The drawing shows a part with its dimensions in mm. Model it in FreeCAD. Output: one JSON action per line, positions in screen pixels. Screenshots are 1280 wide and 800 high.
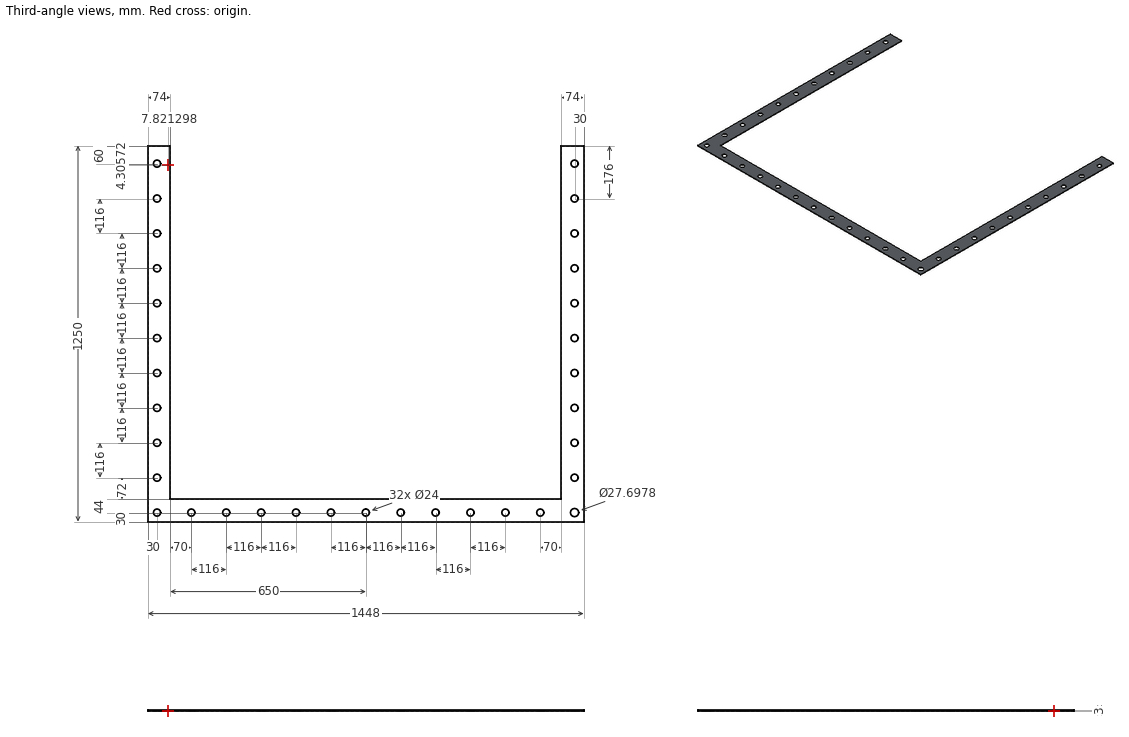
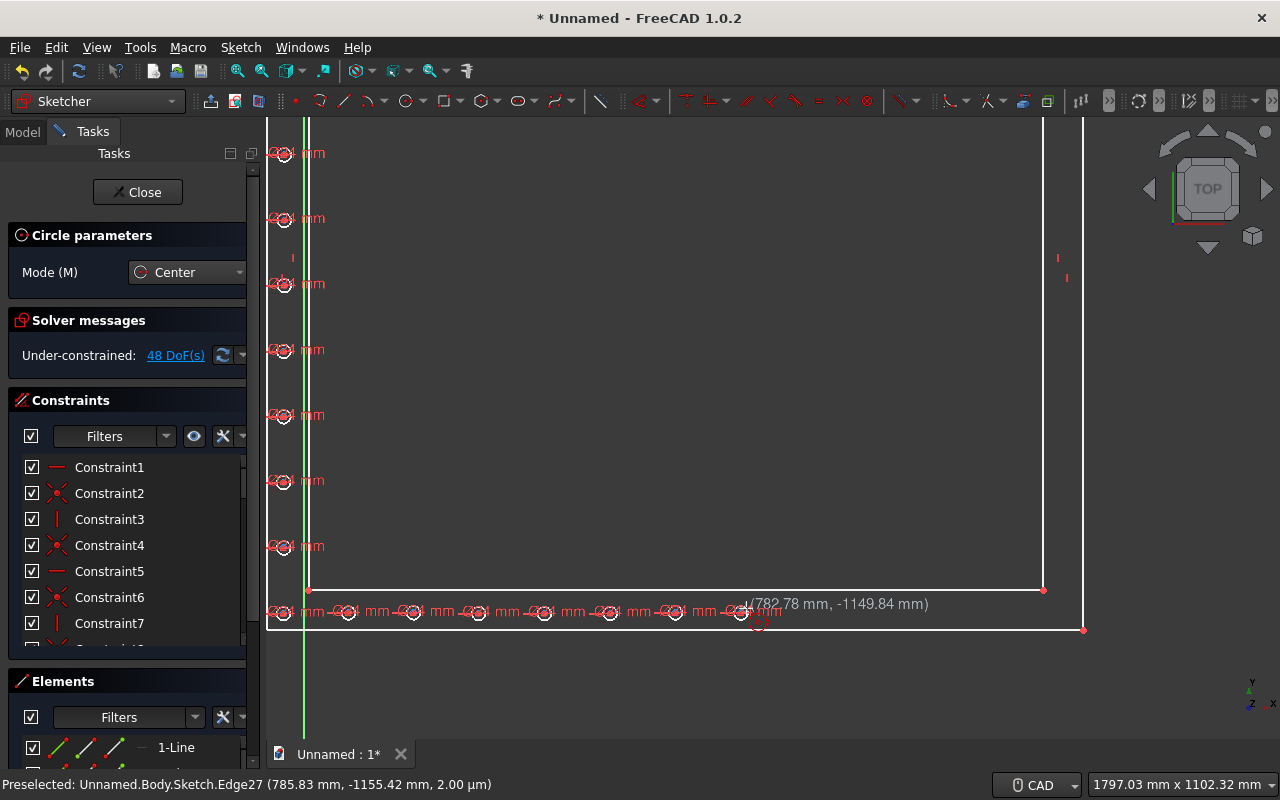
{"action": "scroll", "coordinate": [806, 612], "scroll_direction": "up", "scroll_amount": 7}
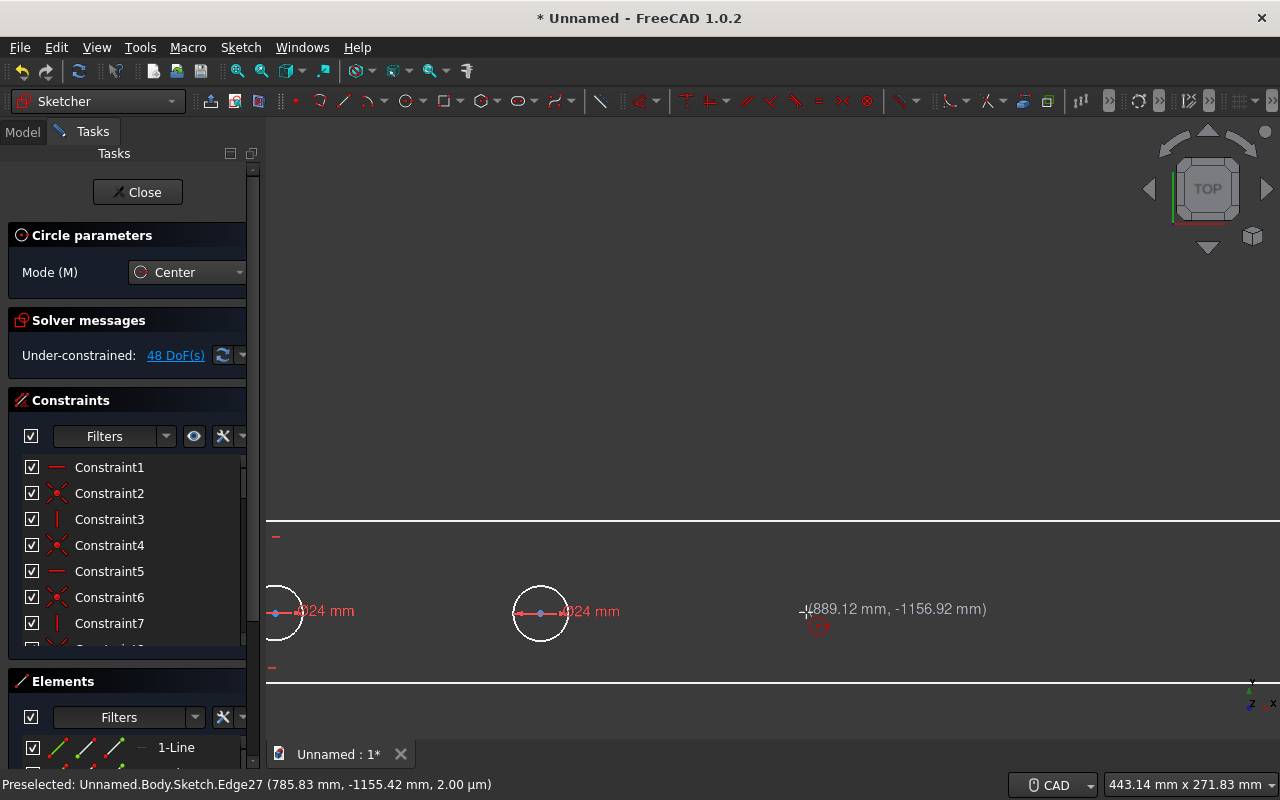
{"action": "scroll", "coordinate": [772, 612], "scroll_direction": "down", "scroll_amount": 10}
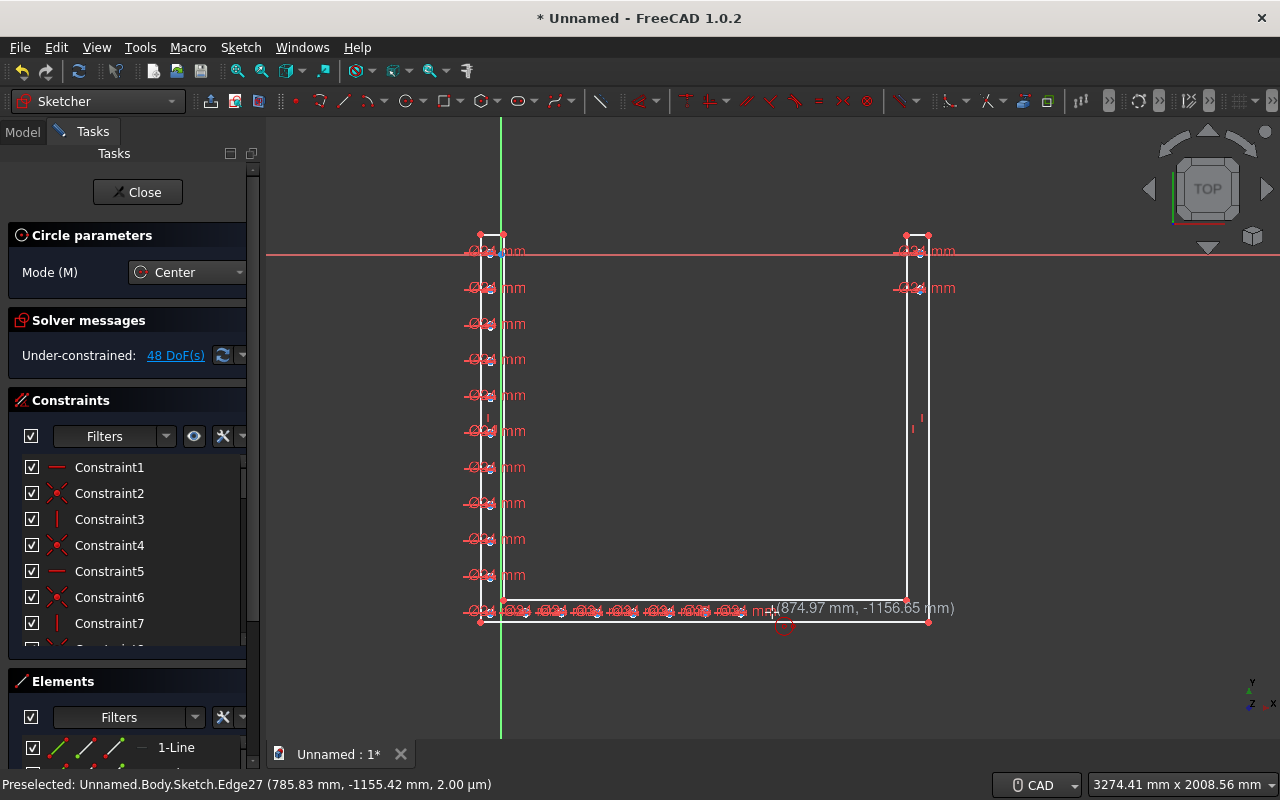
{"action": "scroll", "coordinate": [777, 613], "scroll_direction": "up", "scroll_amount": 3}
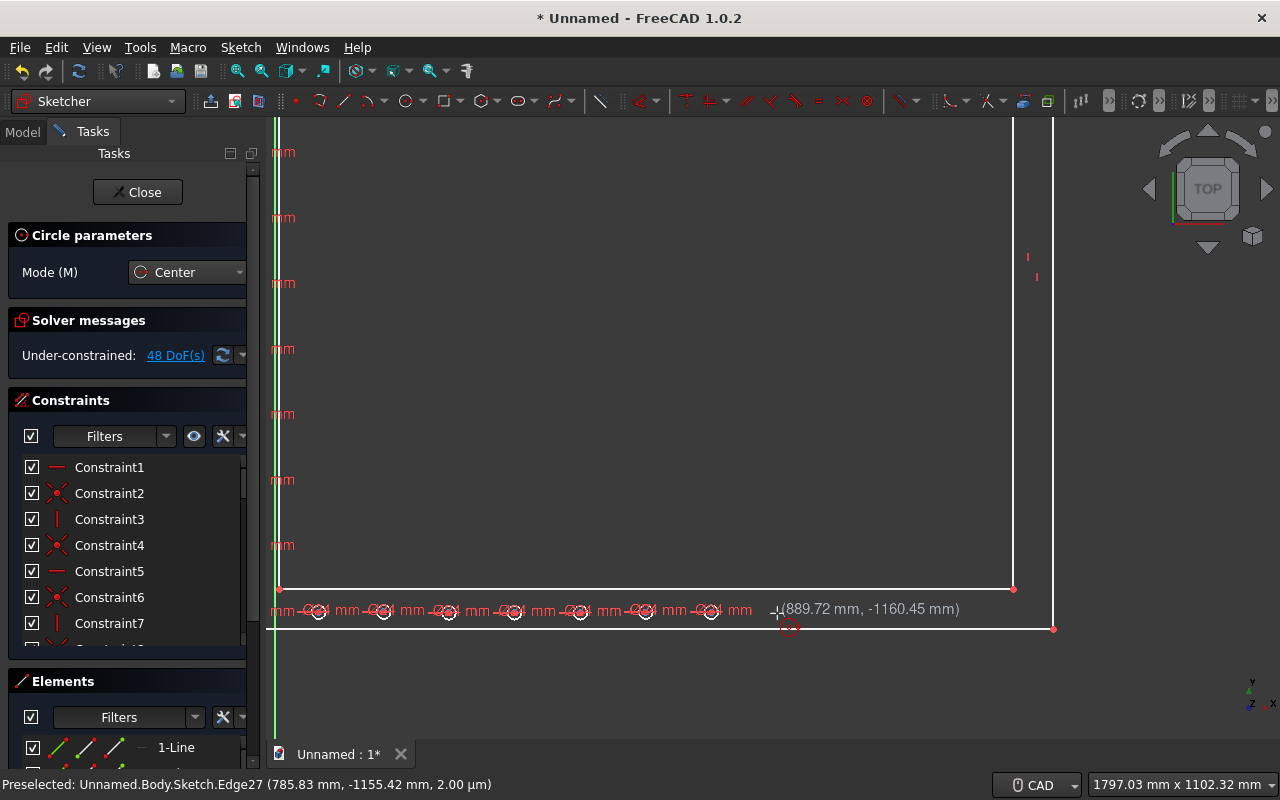
{"action": "left_click", "coordinate": [777, 611]}
{"action": "mouse_move", "coordinate": [781, 607]}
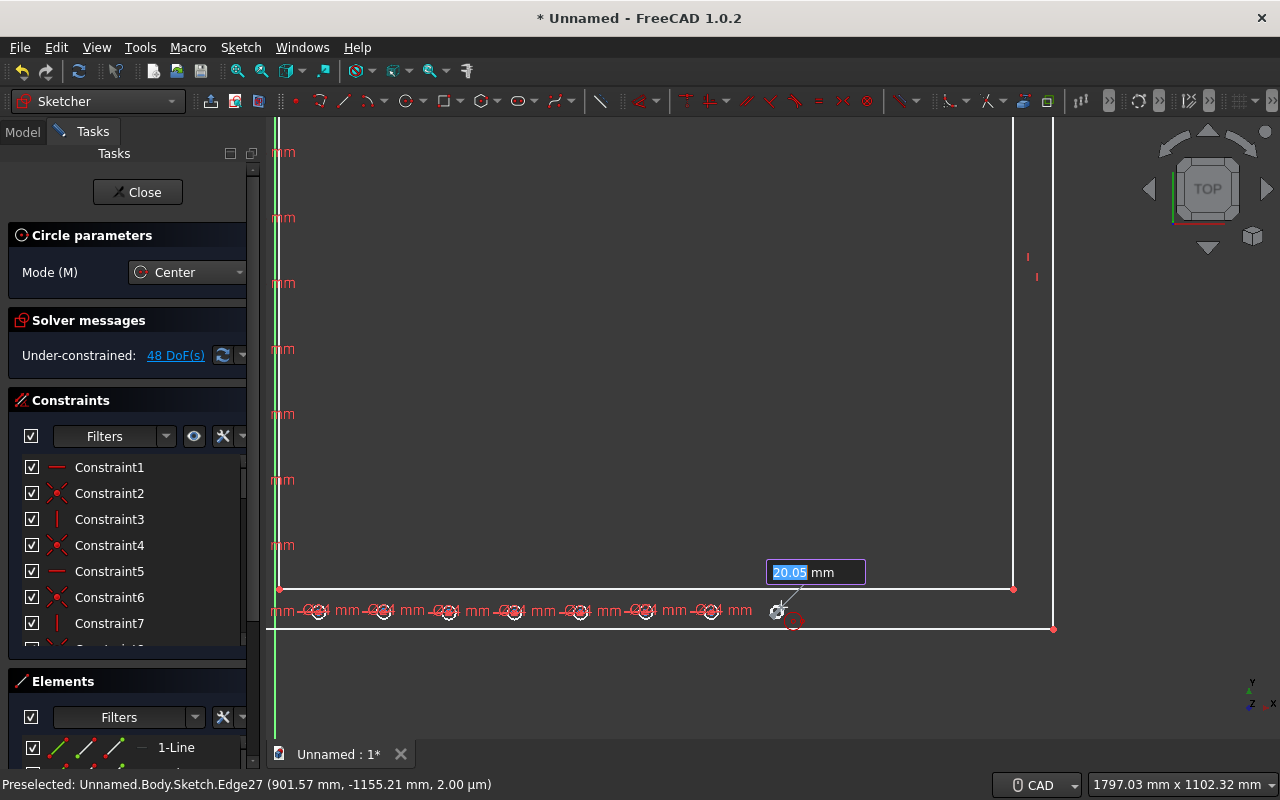
{"action": "type", "text": "24"}
{"action": "key", "text": "Return"}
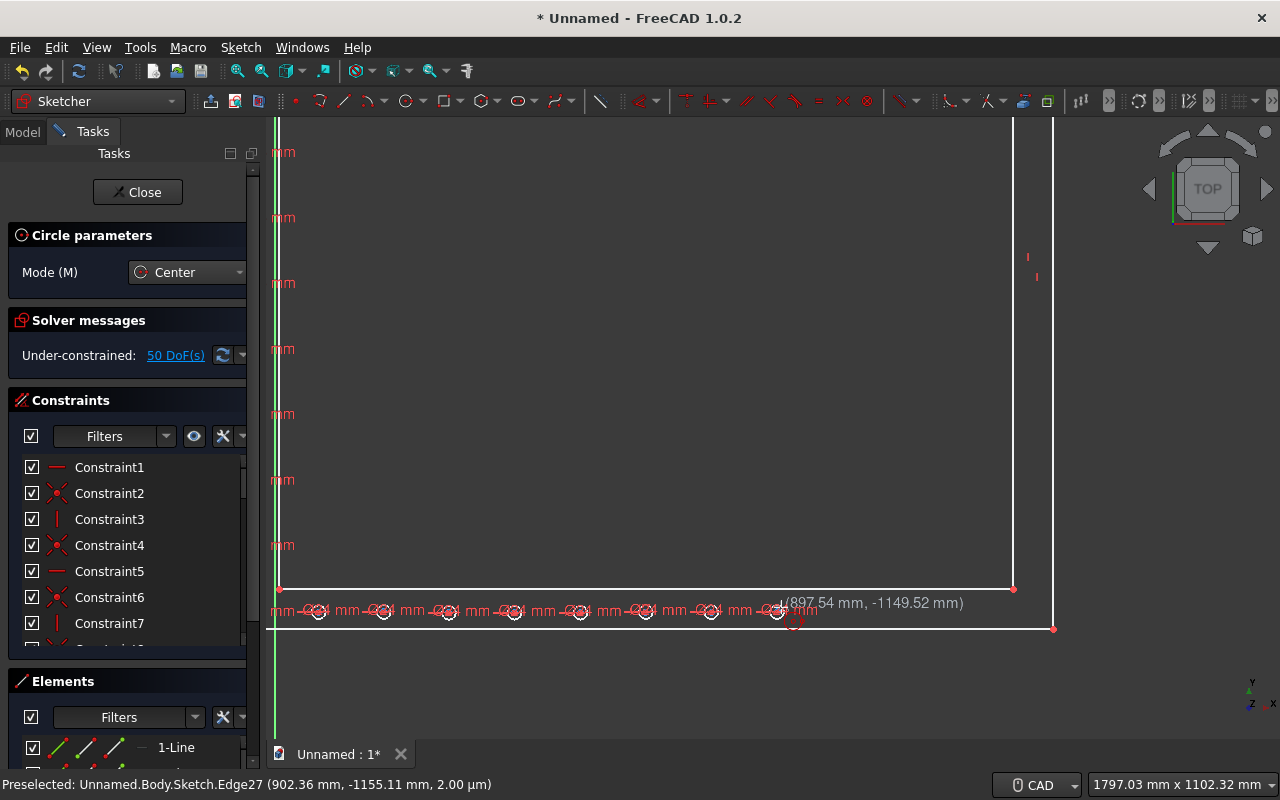
{"action": "scroll", "coordinate": [842, 611], "scroll_direction": "up", "scroll_amount": 7}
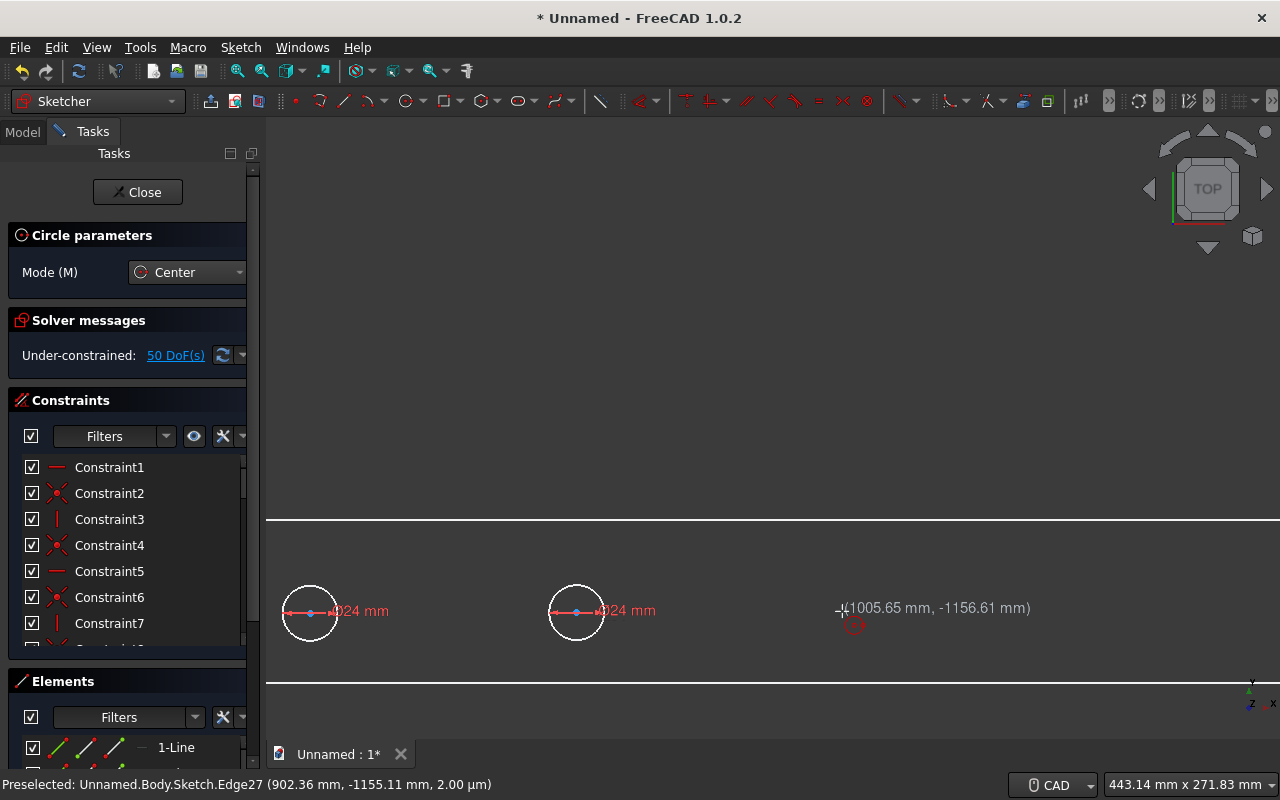
{"action": "scroll", "coordinate": [808, 613], "scroll_direction": "down", "scroll_amount": 10}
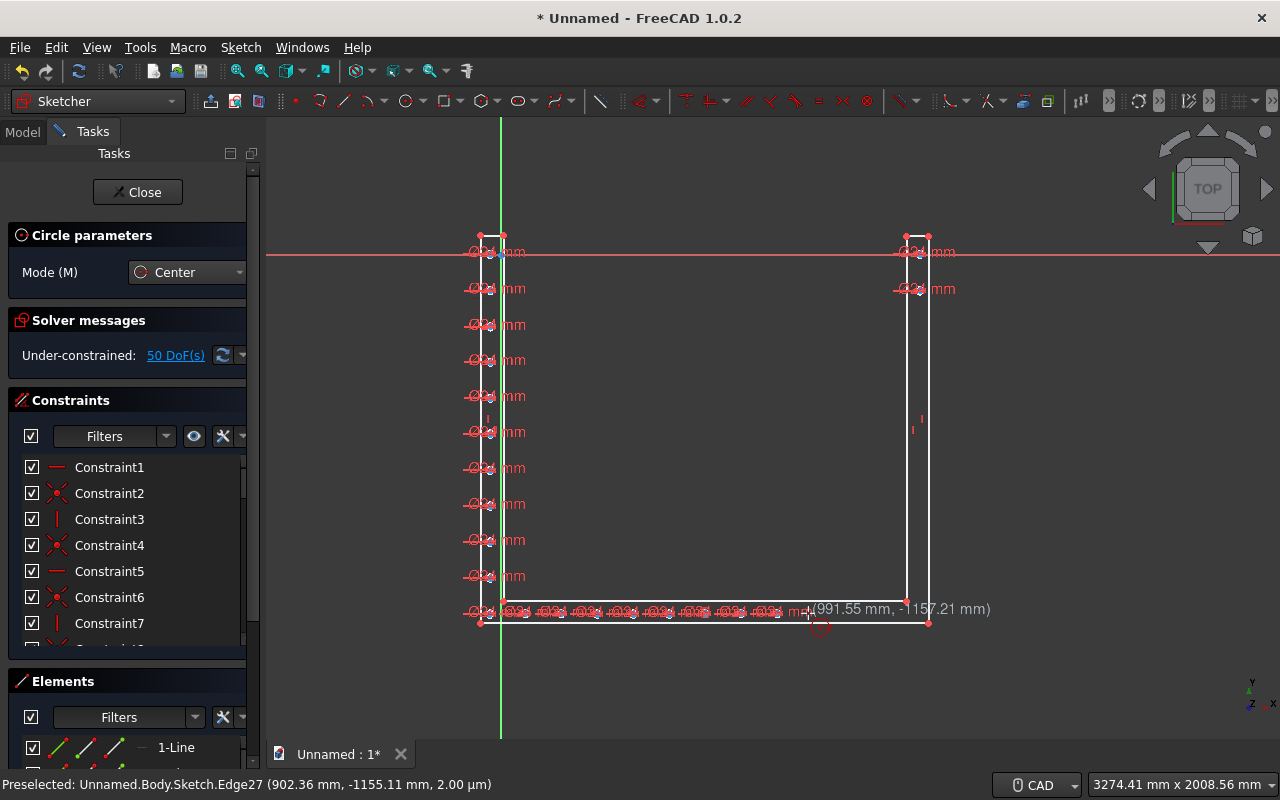
{"action": "scroll", "coordinate": [813, 613], "scroll_direction": "up", "scroll_amount": 3}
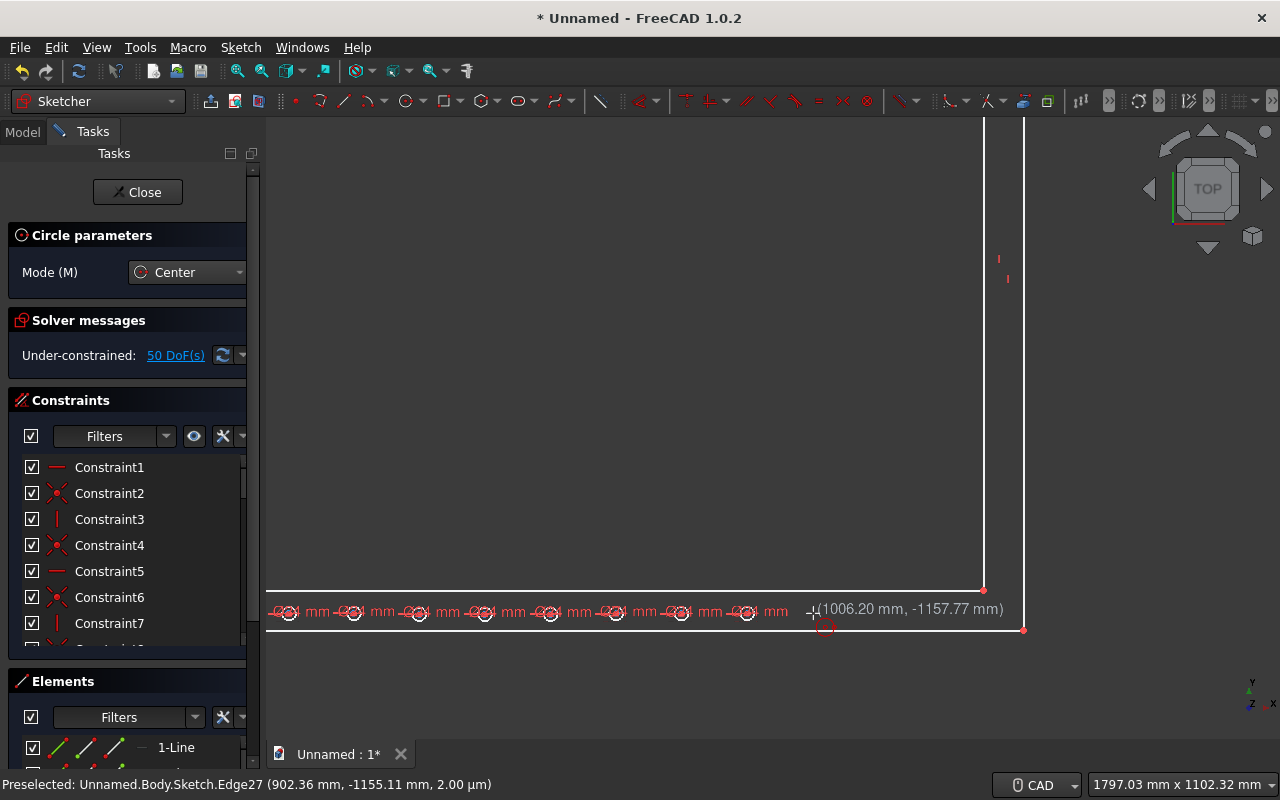
{"action": "left_click", "coordinate": [812, 613]}
{"action": "mouse_move", "coordinate": [817, 608]}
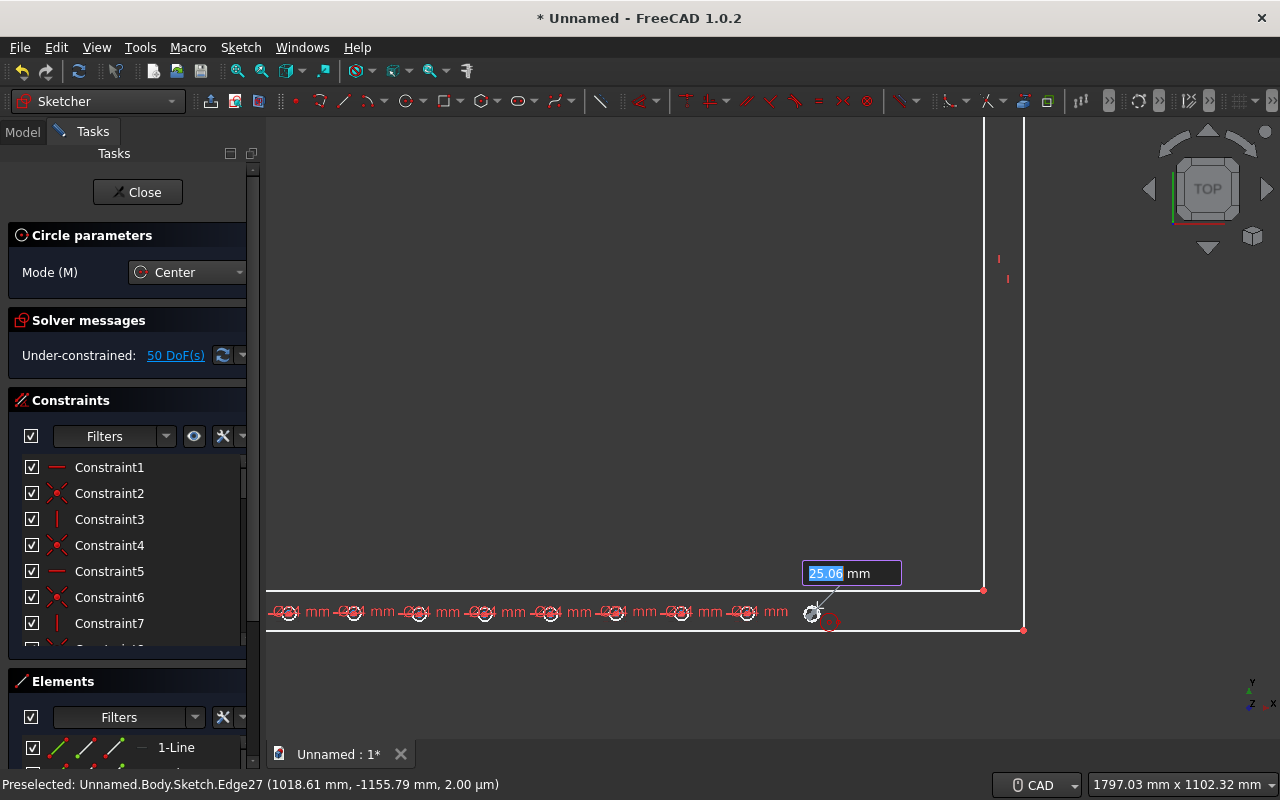
{"action": "type", "text": "24"}
{"action": "key", "text": "Return"}